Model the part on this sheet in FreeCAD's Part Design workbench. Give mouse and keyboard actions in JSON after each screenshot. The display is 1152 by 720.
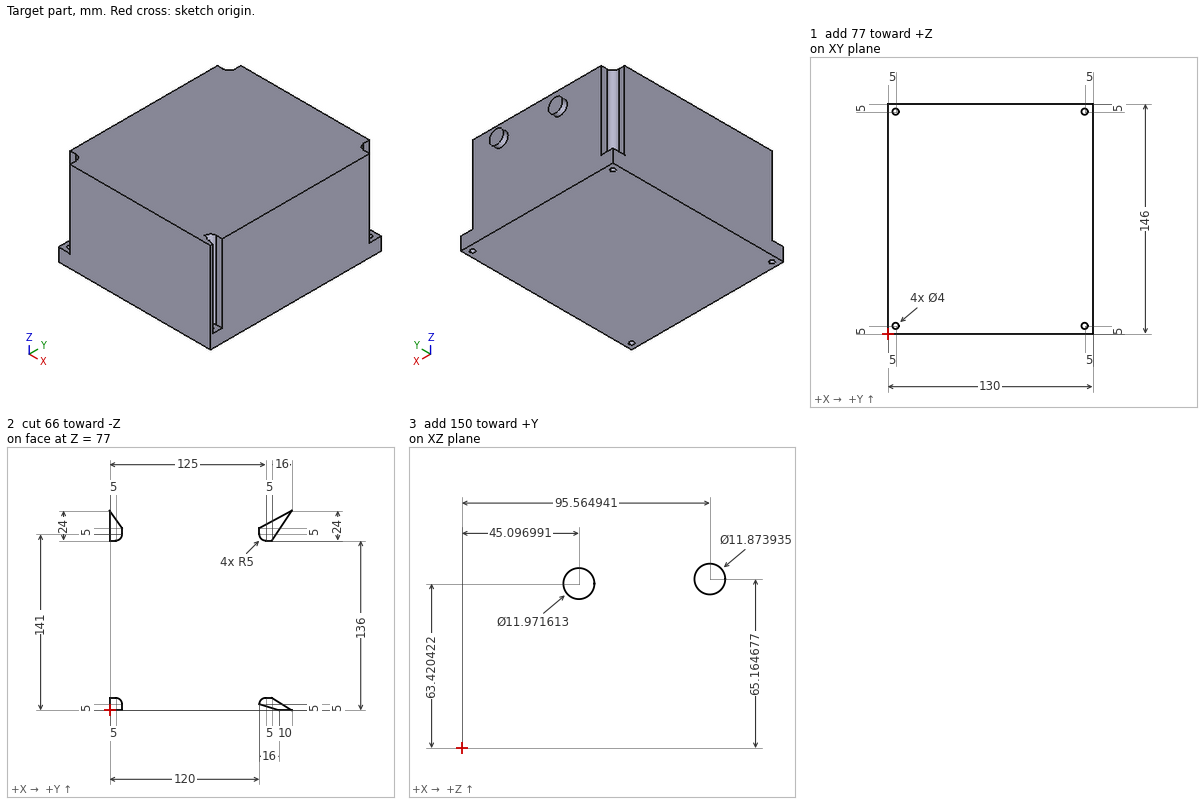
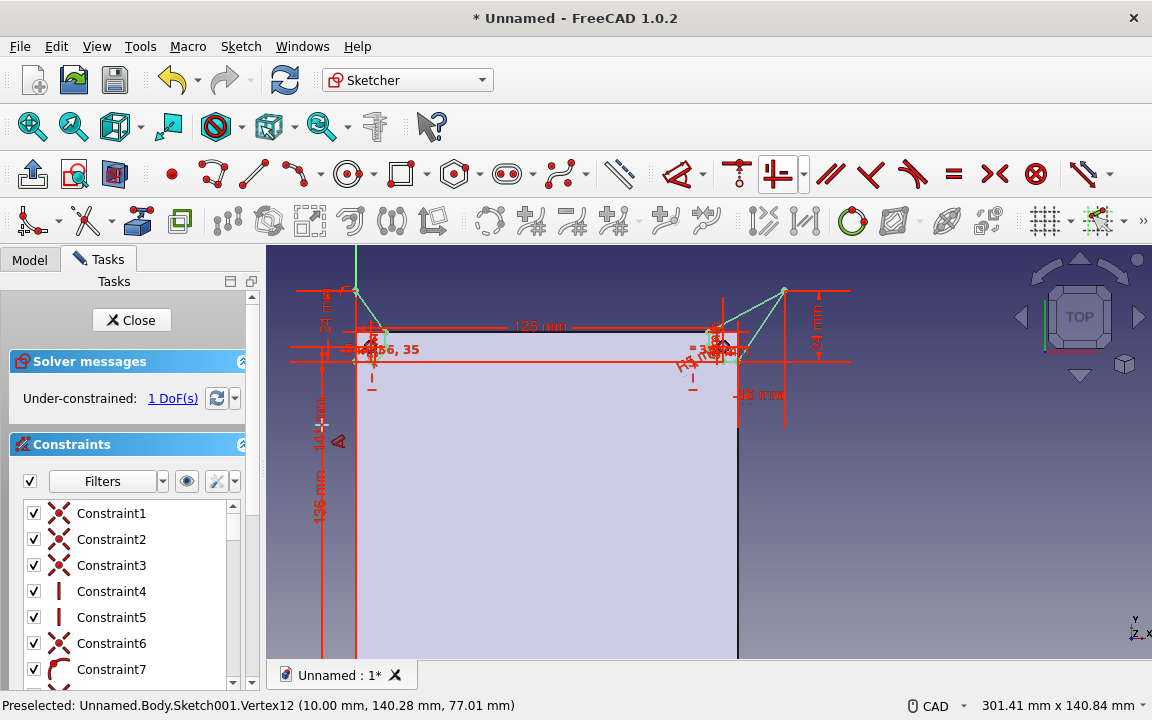
{"action": "scroll", "coordinate": [726, 362], "scroll_direction": "down", "scroll_amount": 3}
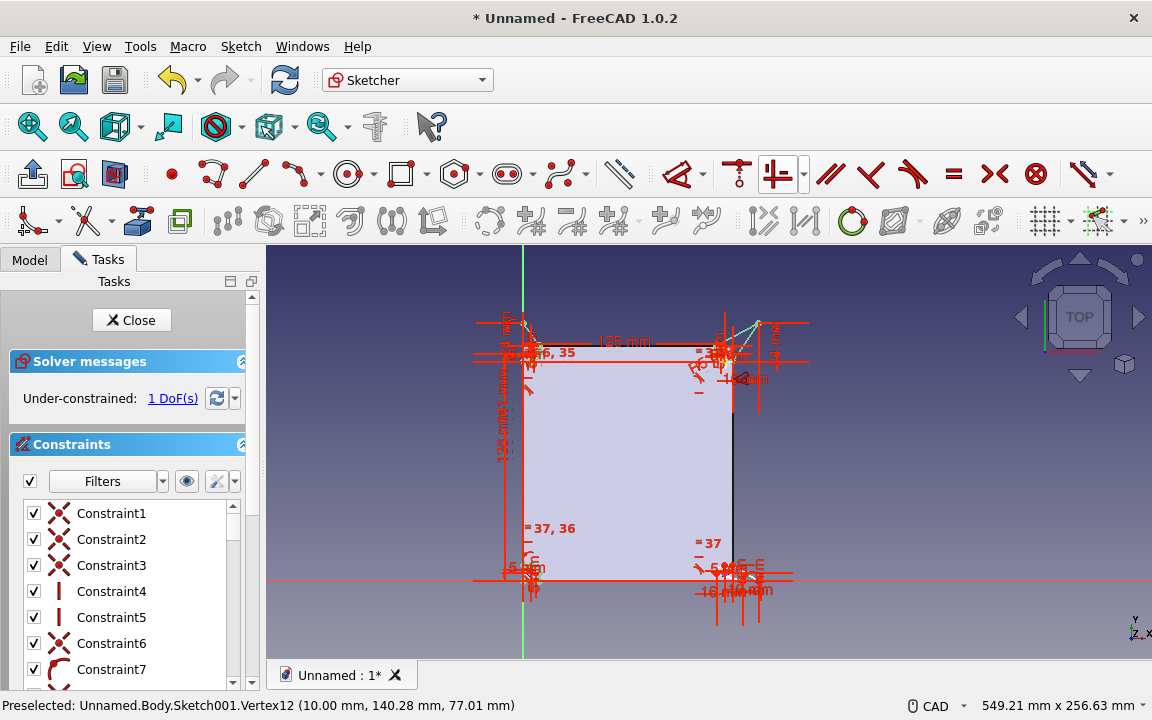
{"action": "scroll", "coordinate": [717, 573], "scroll_direction": "up", "scroll_amount": 3}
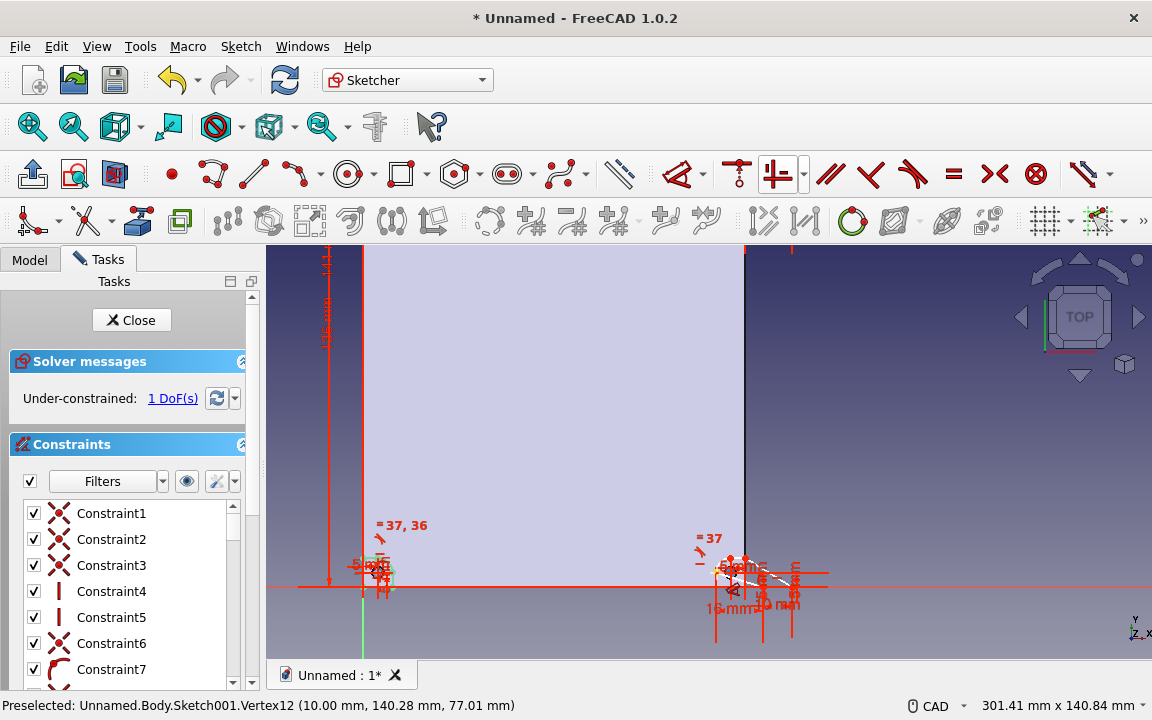
{"action": "left_click", "coordinate": [716, 573]}
{"action": "left_click", "coordinate": [540, 621]}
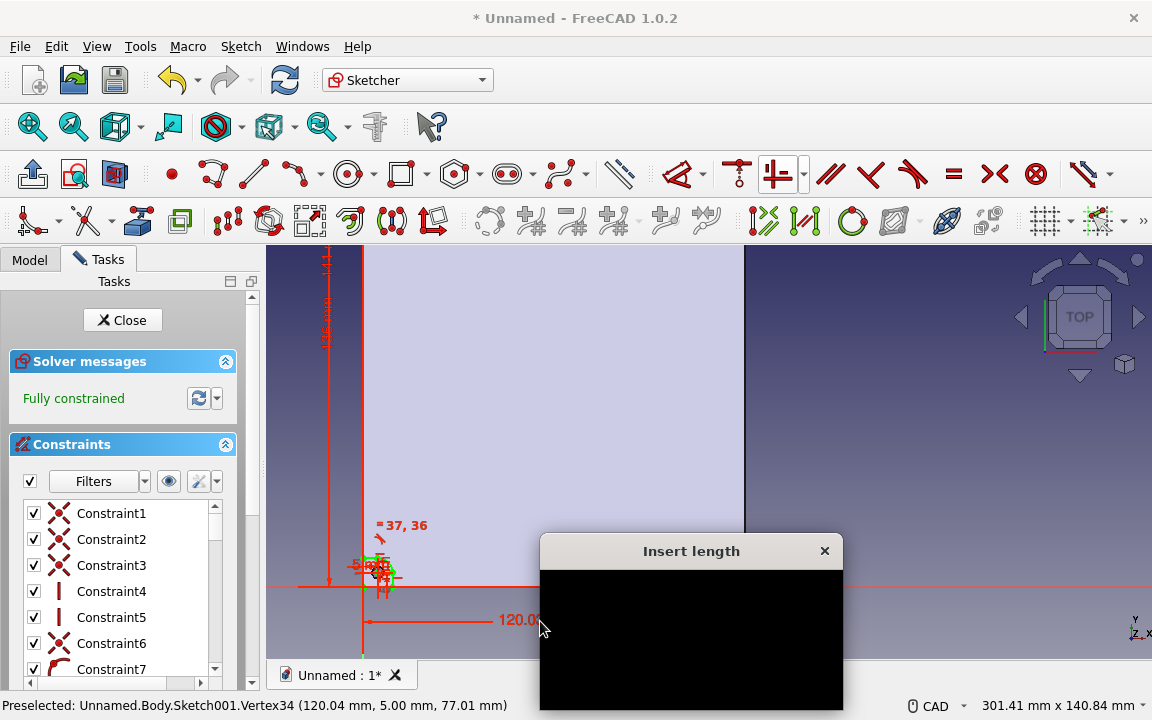
{"action": "type", "text": "120"}
{"action": "key", "text": "Return"}
{"action": "key", "text": "Escape"}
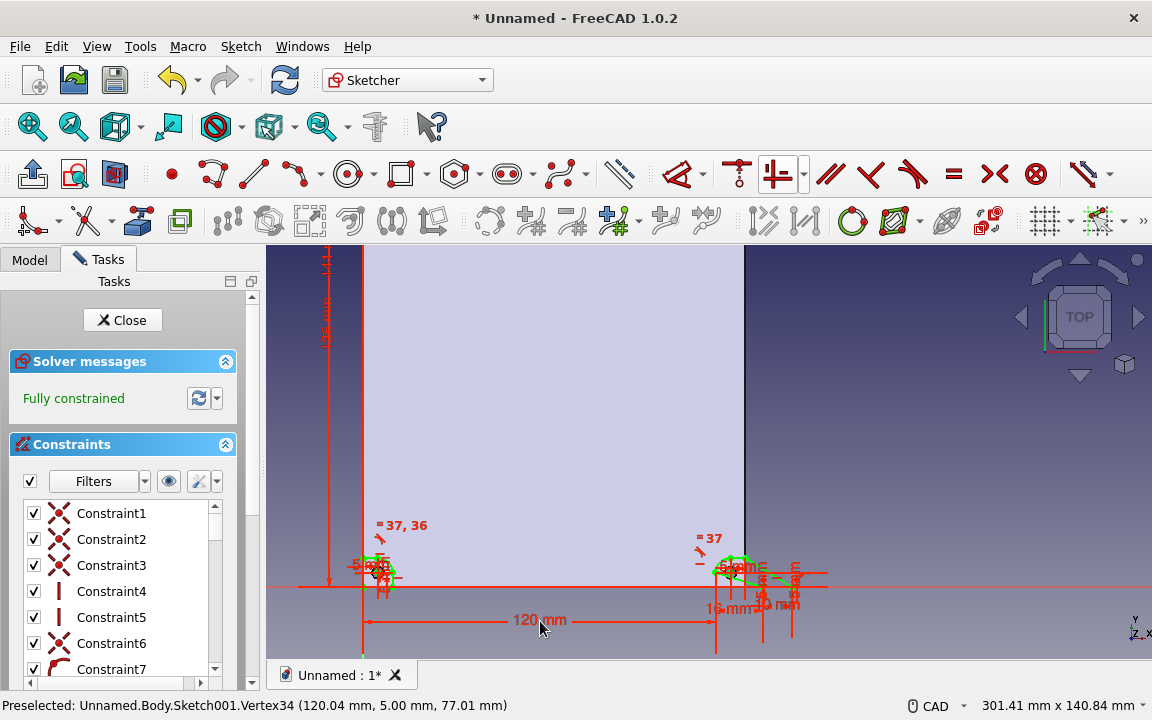
{"action": "left_click", "coordinate": [123, 320]}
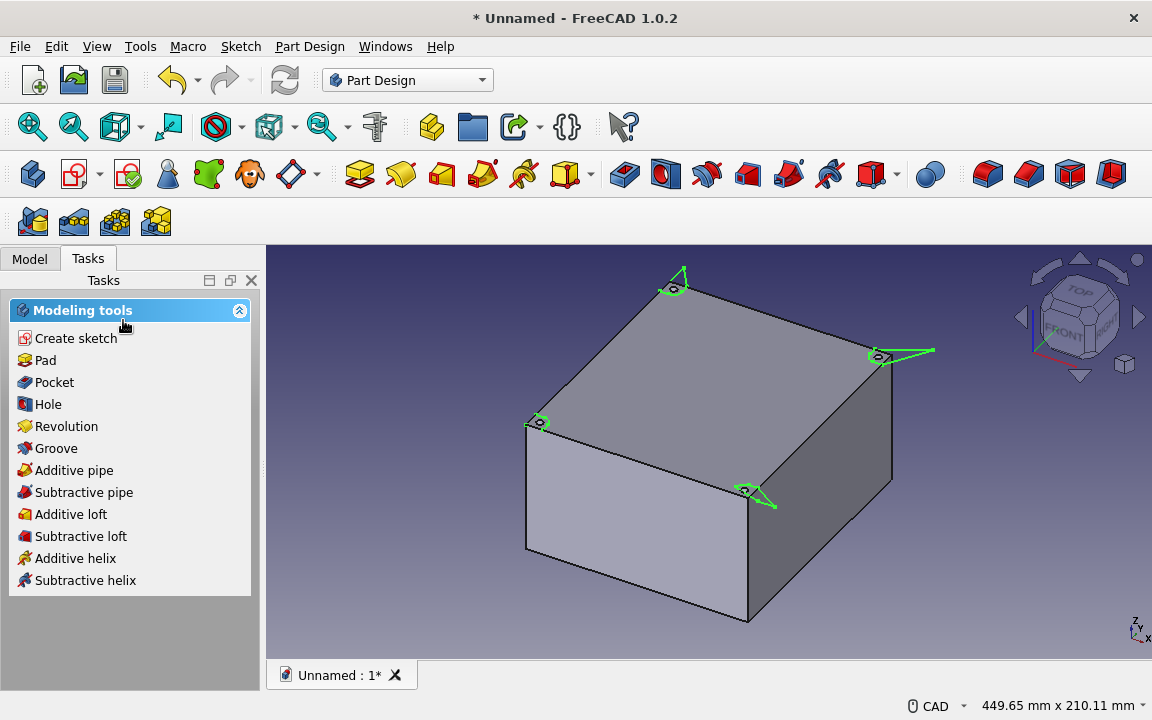
{"action": "left_click", "coordinate": [625, 174]}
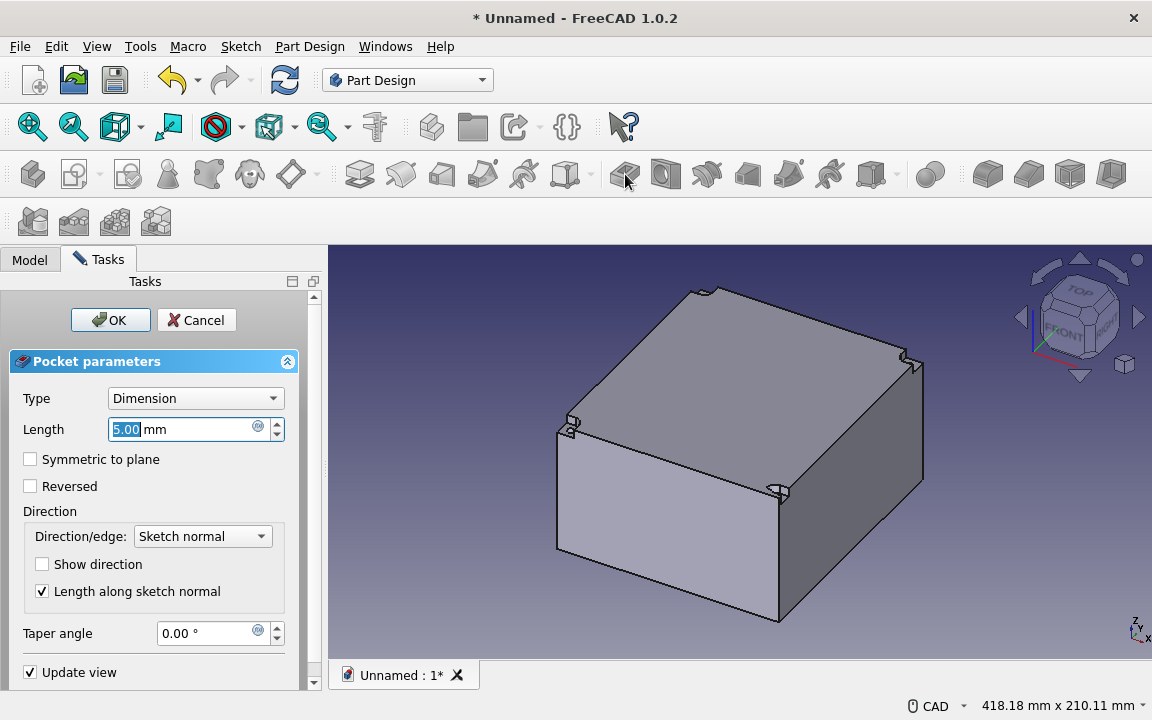
{"action": "type", "text": "66"}
{"action": "key", "text": "Tab"}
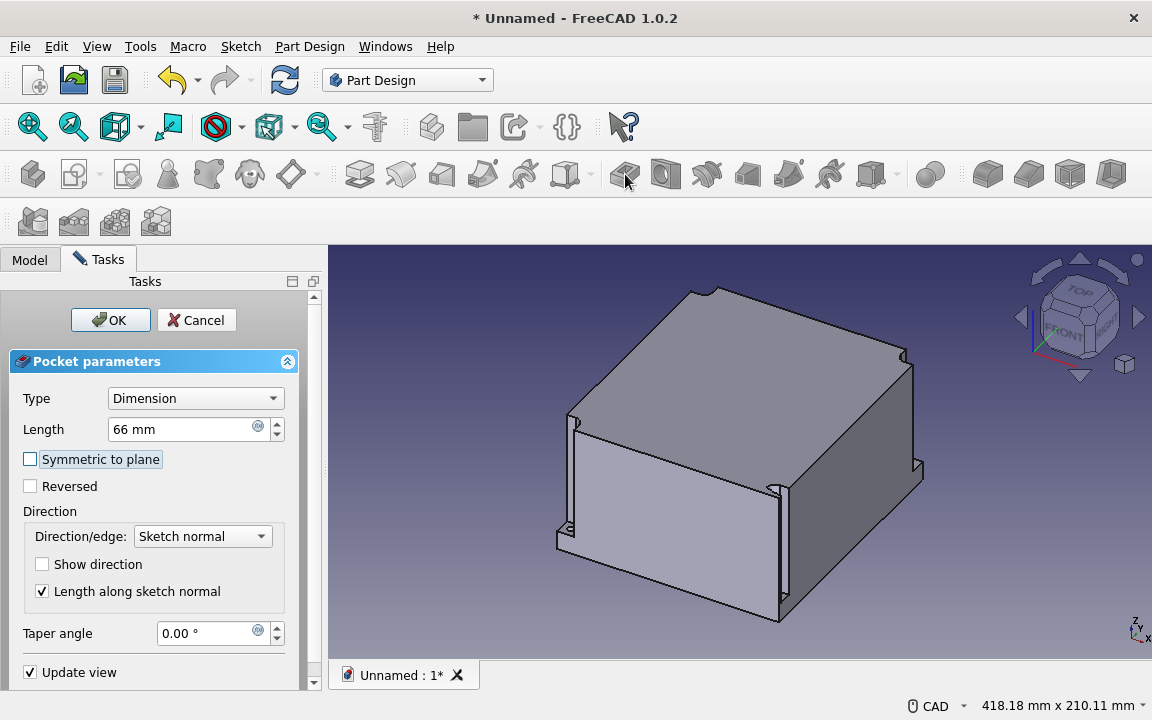
{"action": "left_click", "coordinate": [111, 320]}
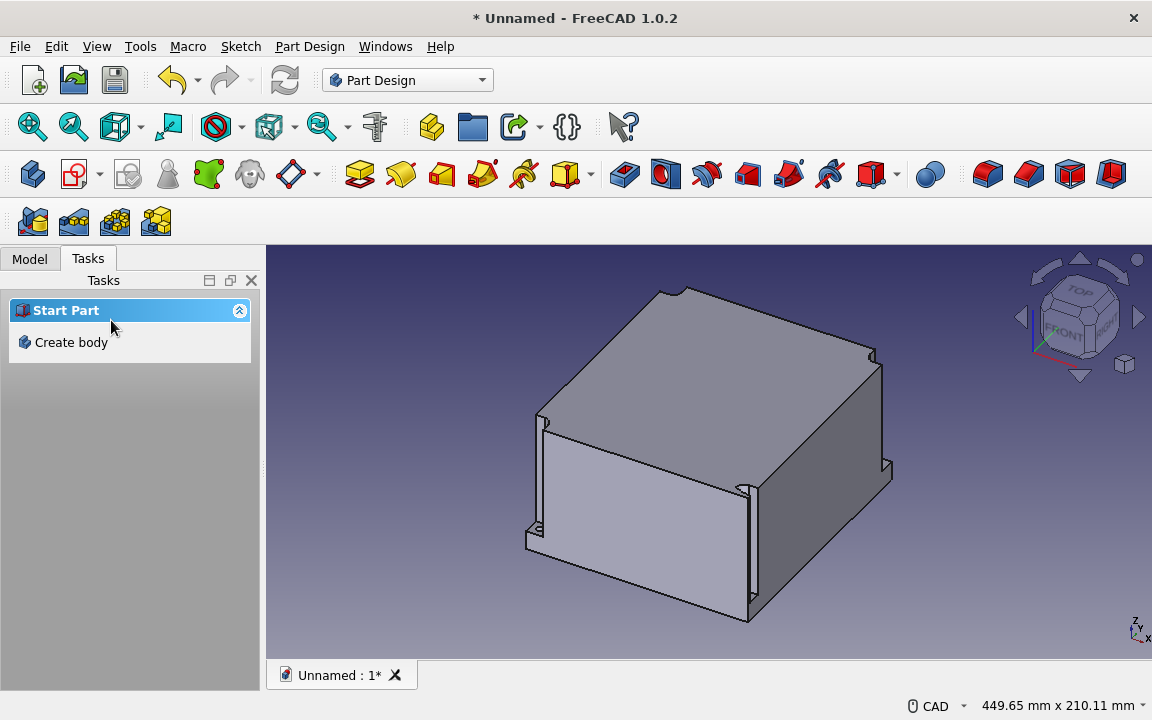
{"action": "left_click", "coordinate": [74, 174]}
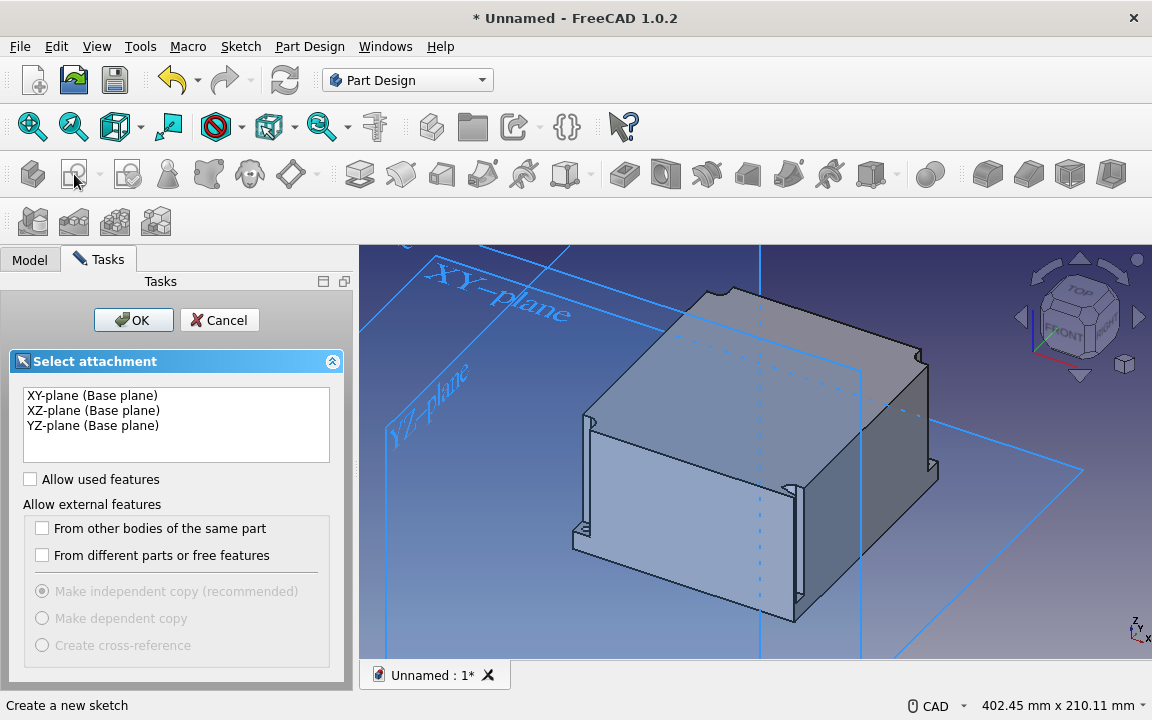
{"action": "left_click", "coordinate": [84, 410]}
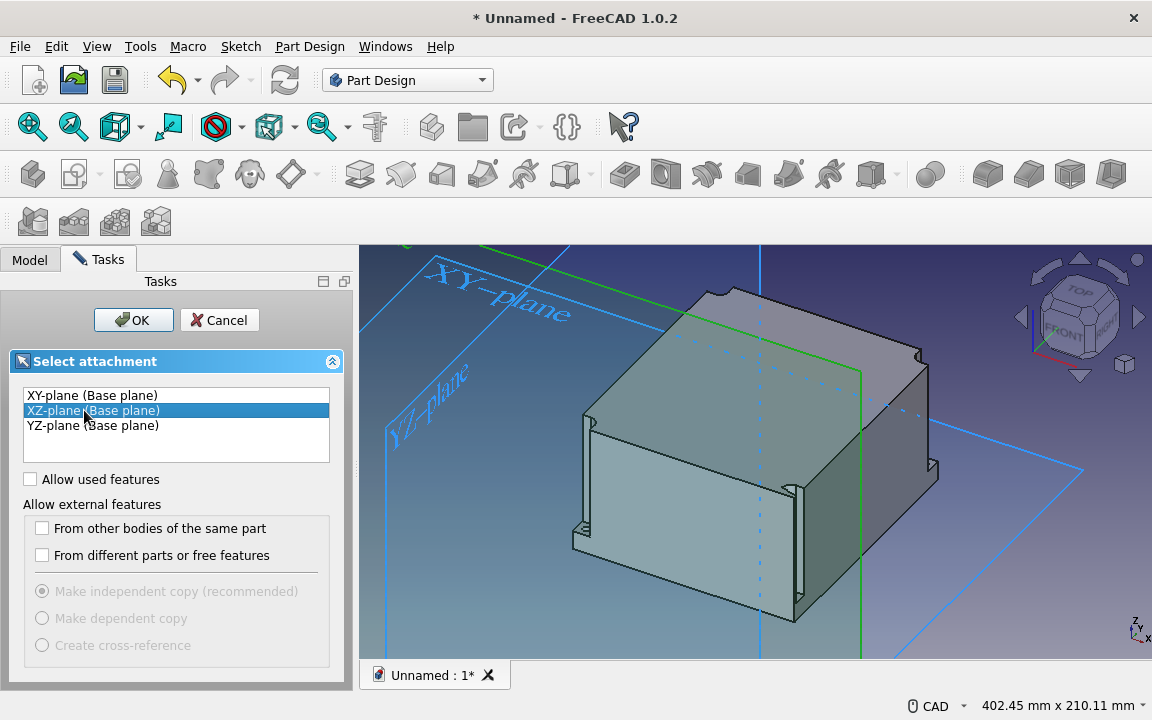
{"action": "left_click", "coordinate": [134, 320]}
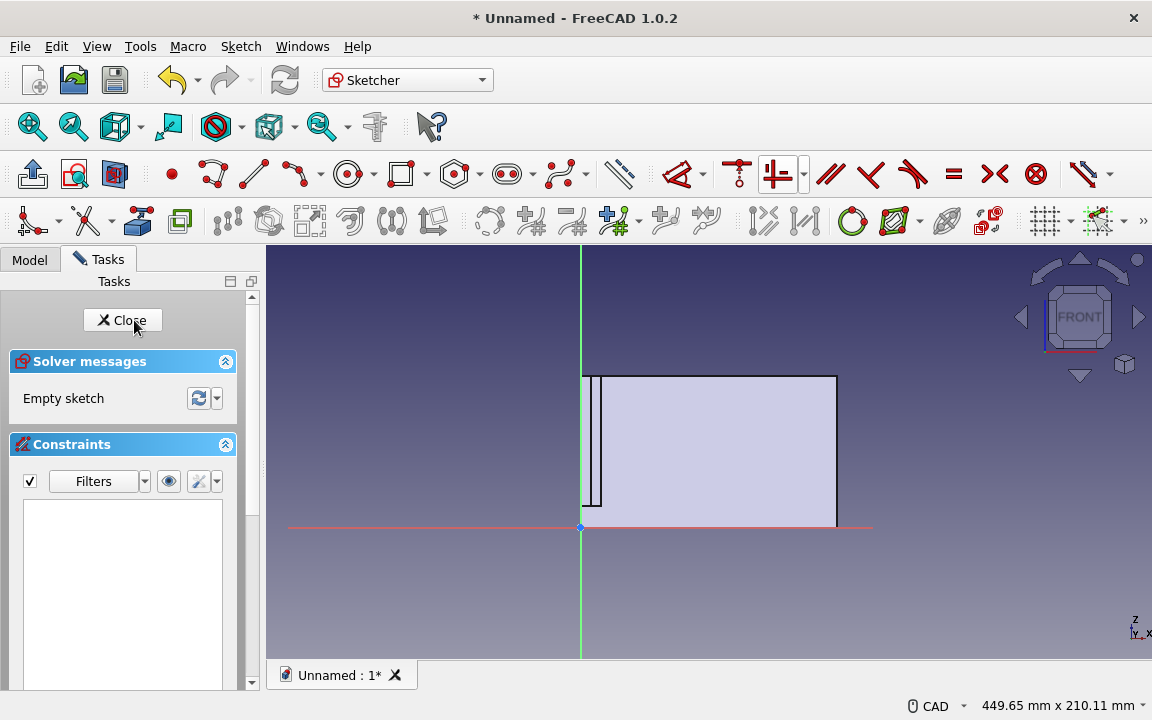
{"action": "scroll", "coordinate": [730, 465], "scroll_direction": "up", "scroll_amount": 3}